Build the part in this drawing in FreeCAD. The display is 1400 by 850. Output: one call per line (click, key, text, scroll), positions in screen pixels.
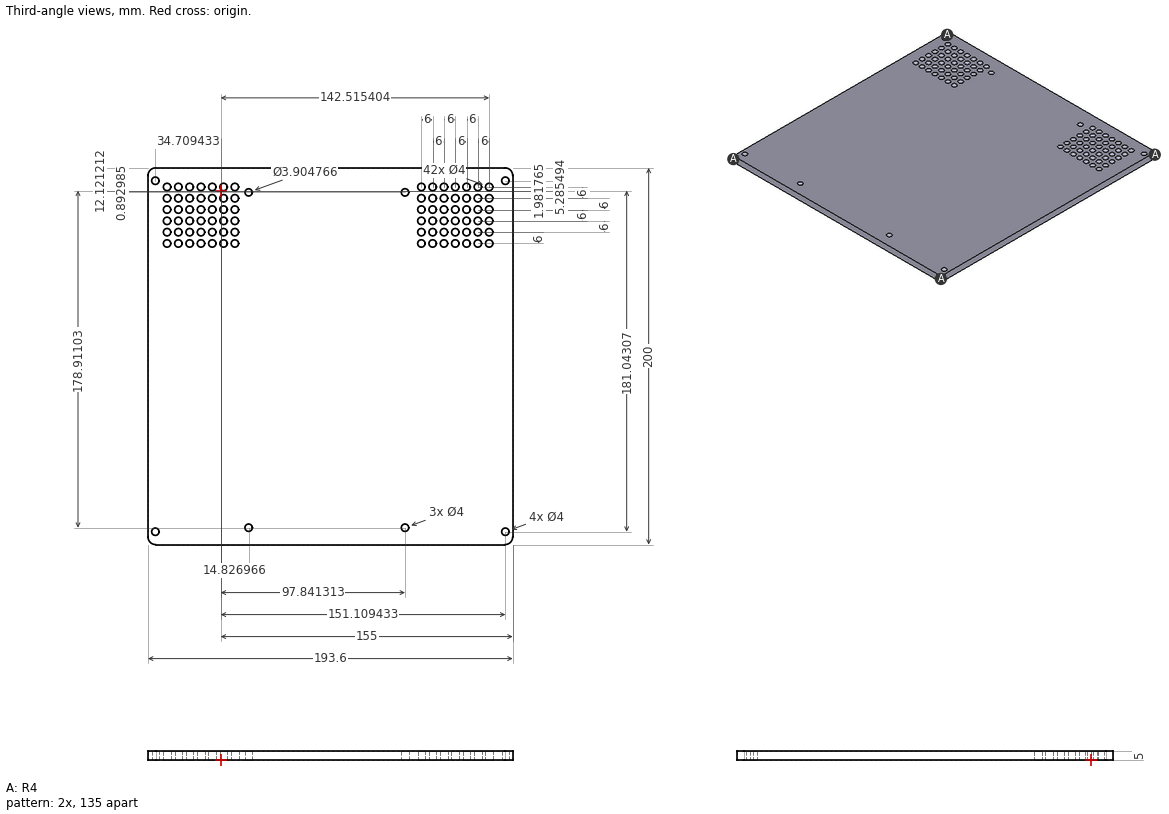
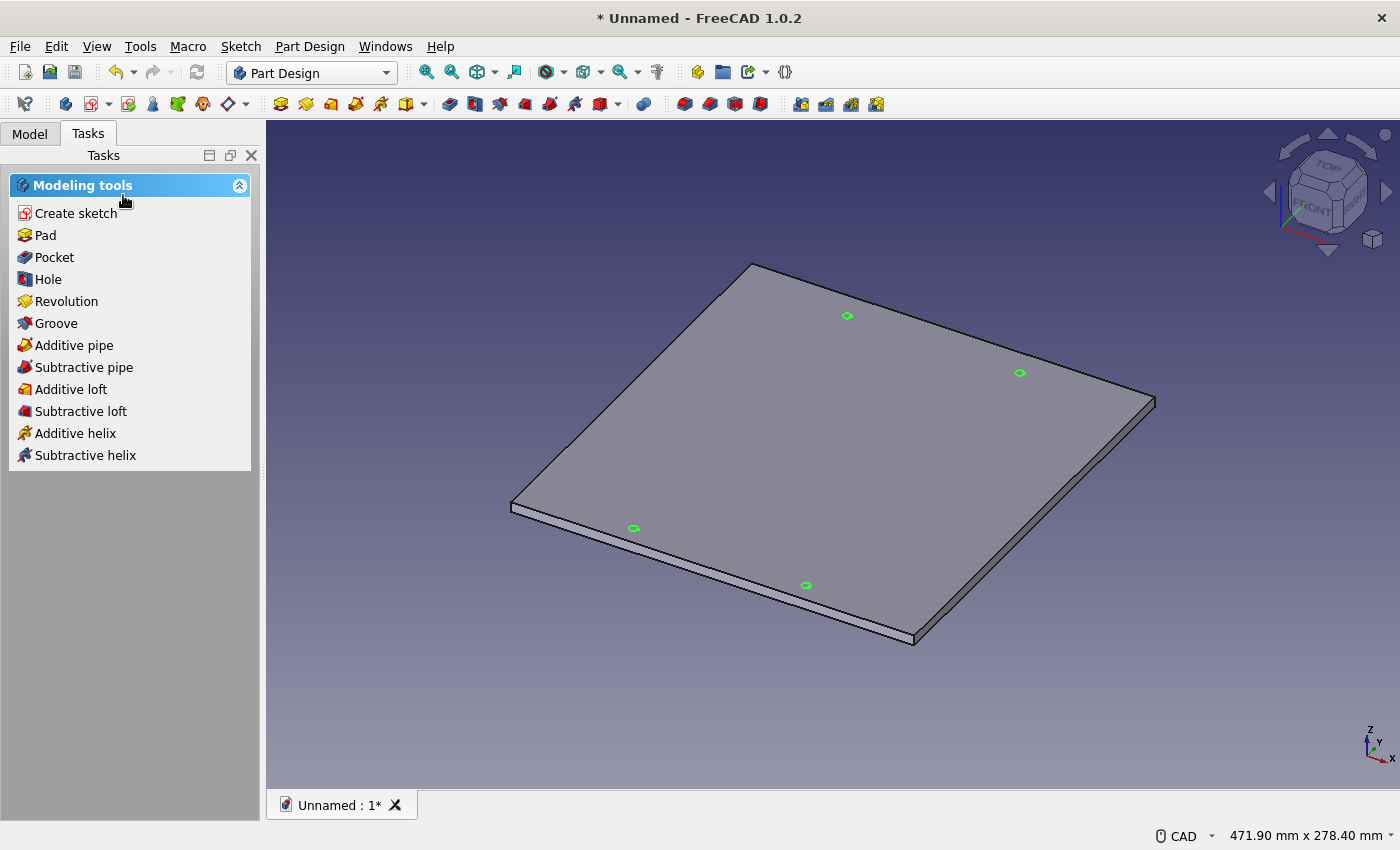
click(450, 104)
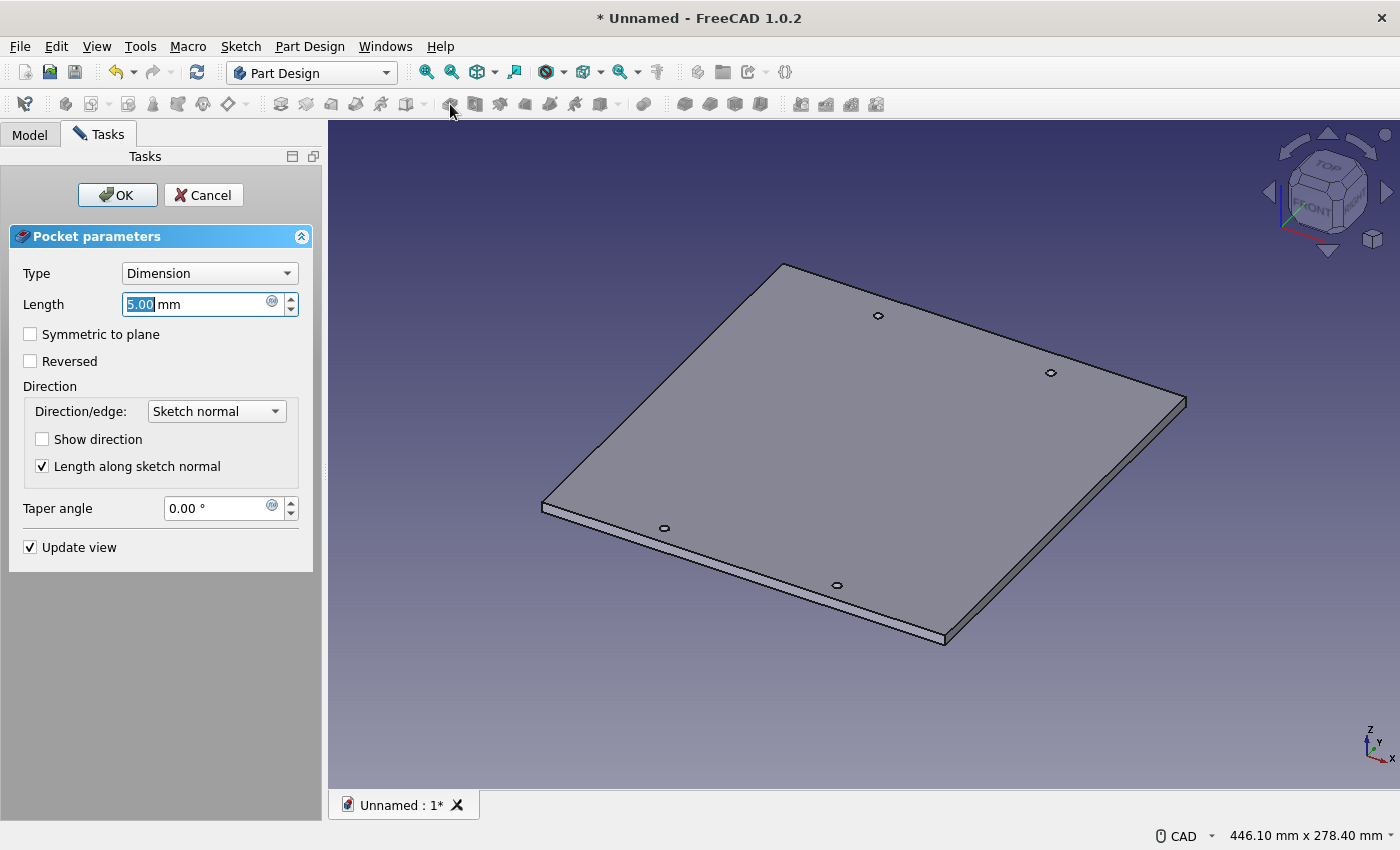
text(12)
key(Tab)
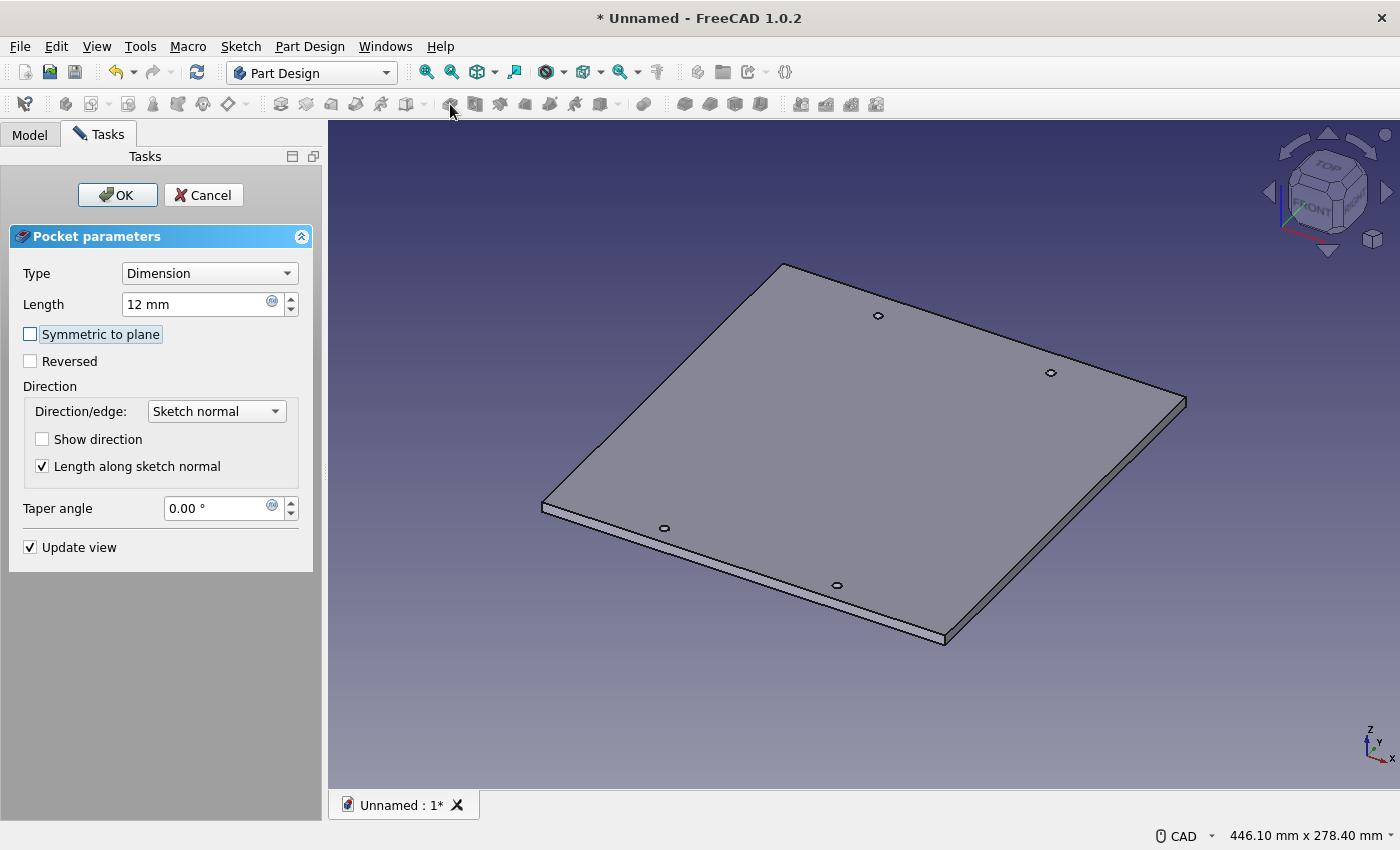
click(118, 195)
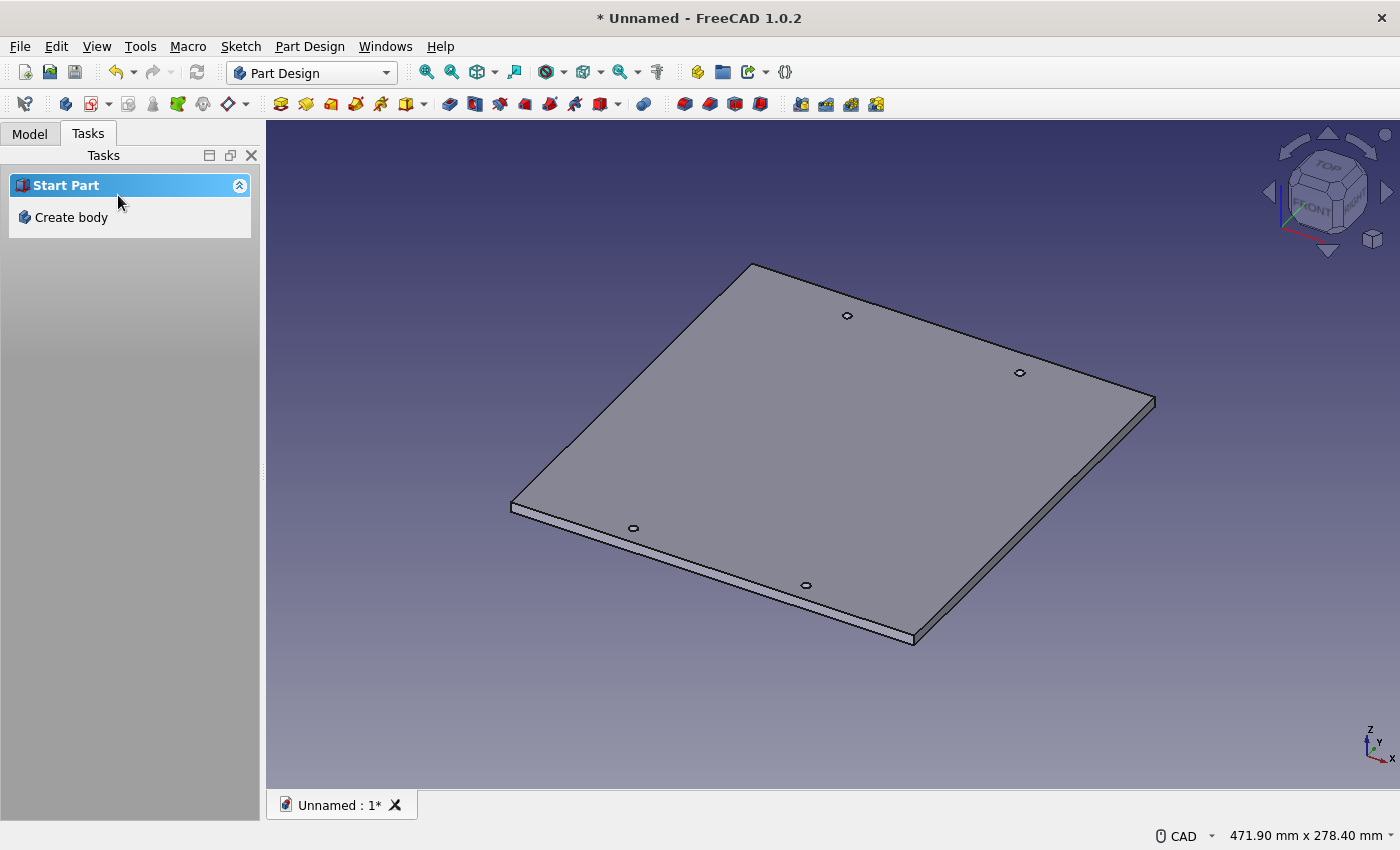
click(833, 449)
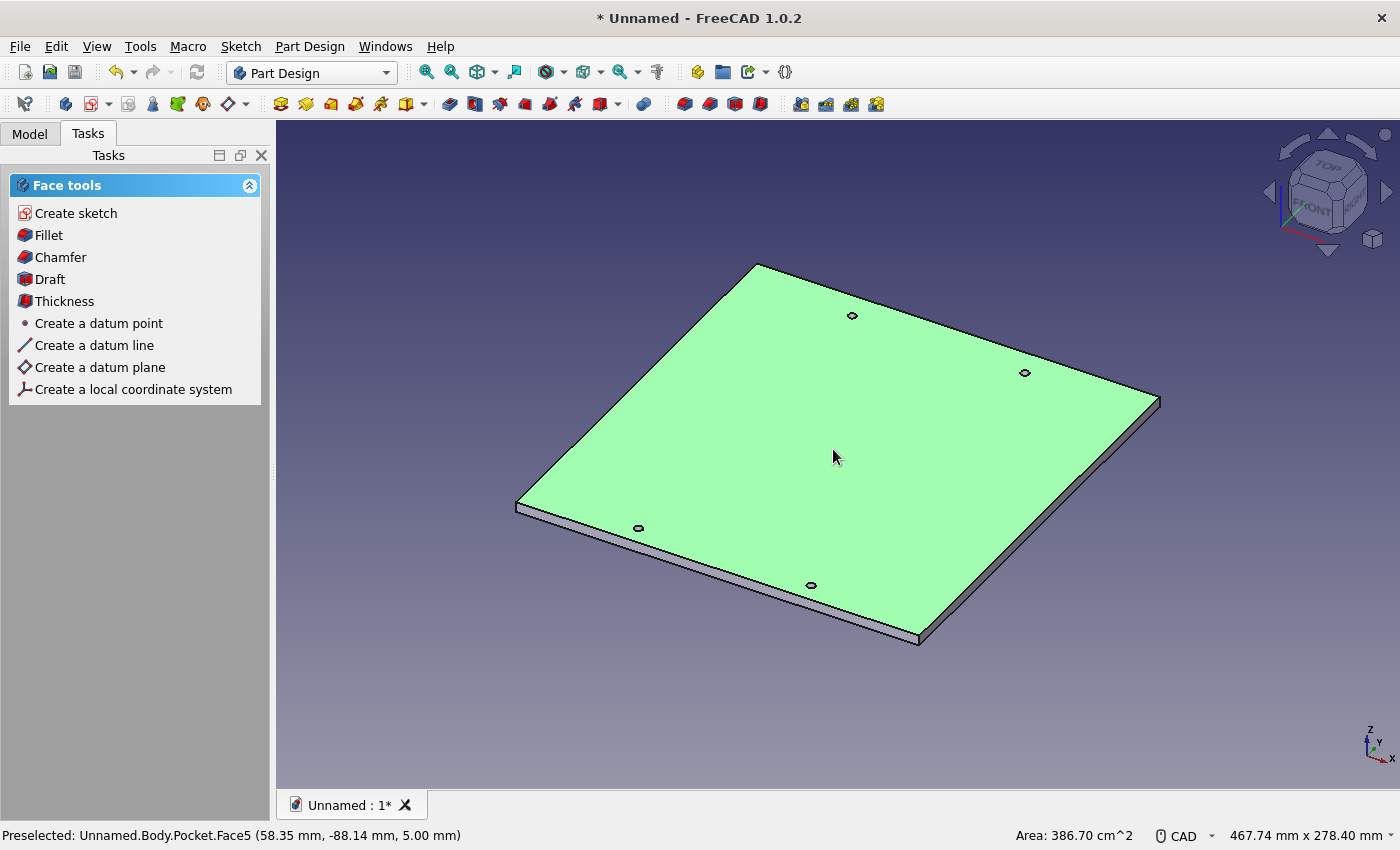
click(90, 104)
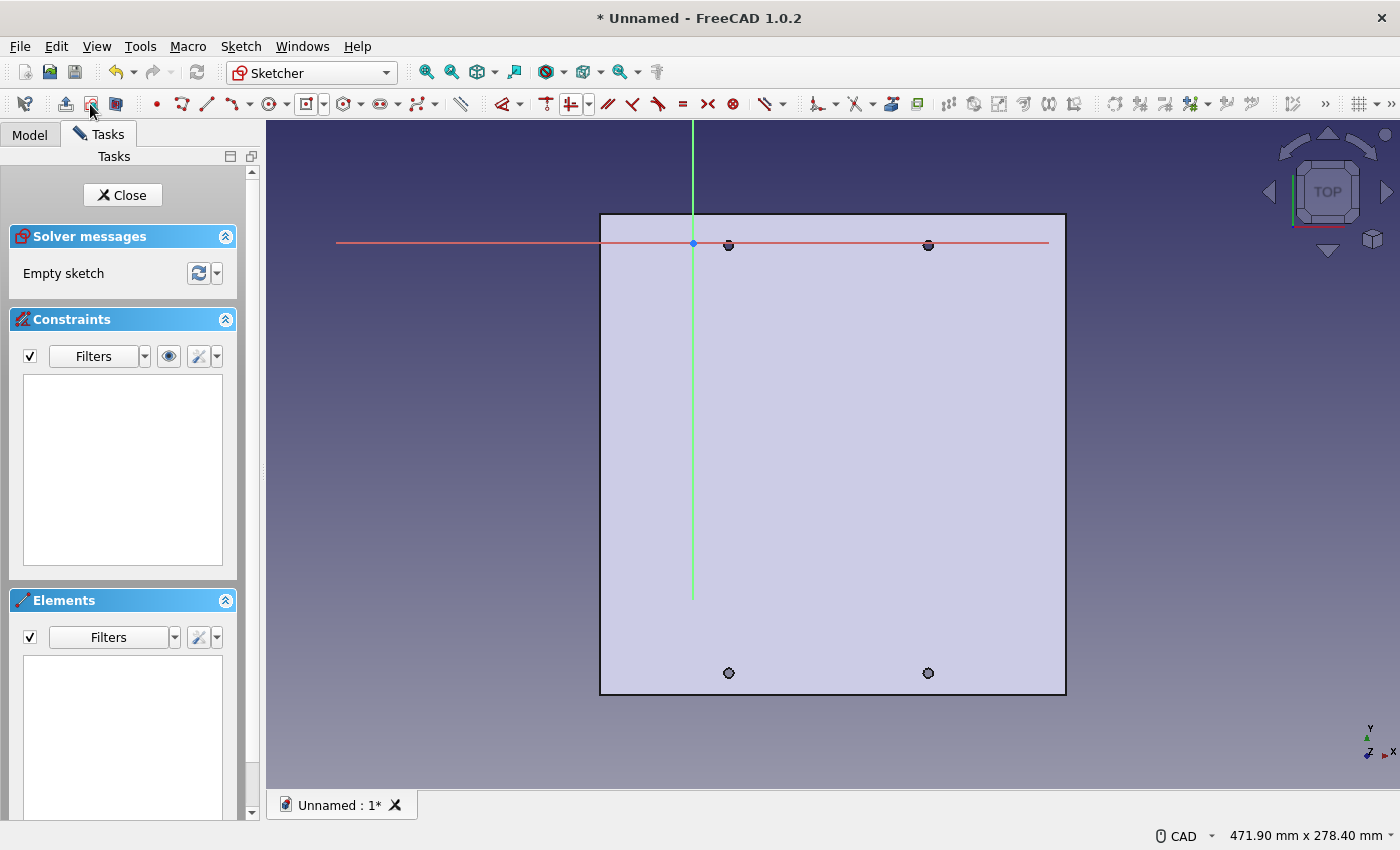
click(268, 104)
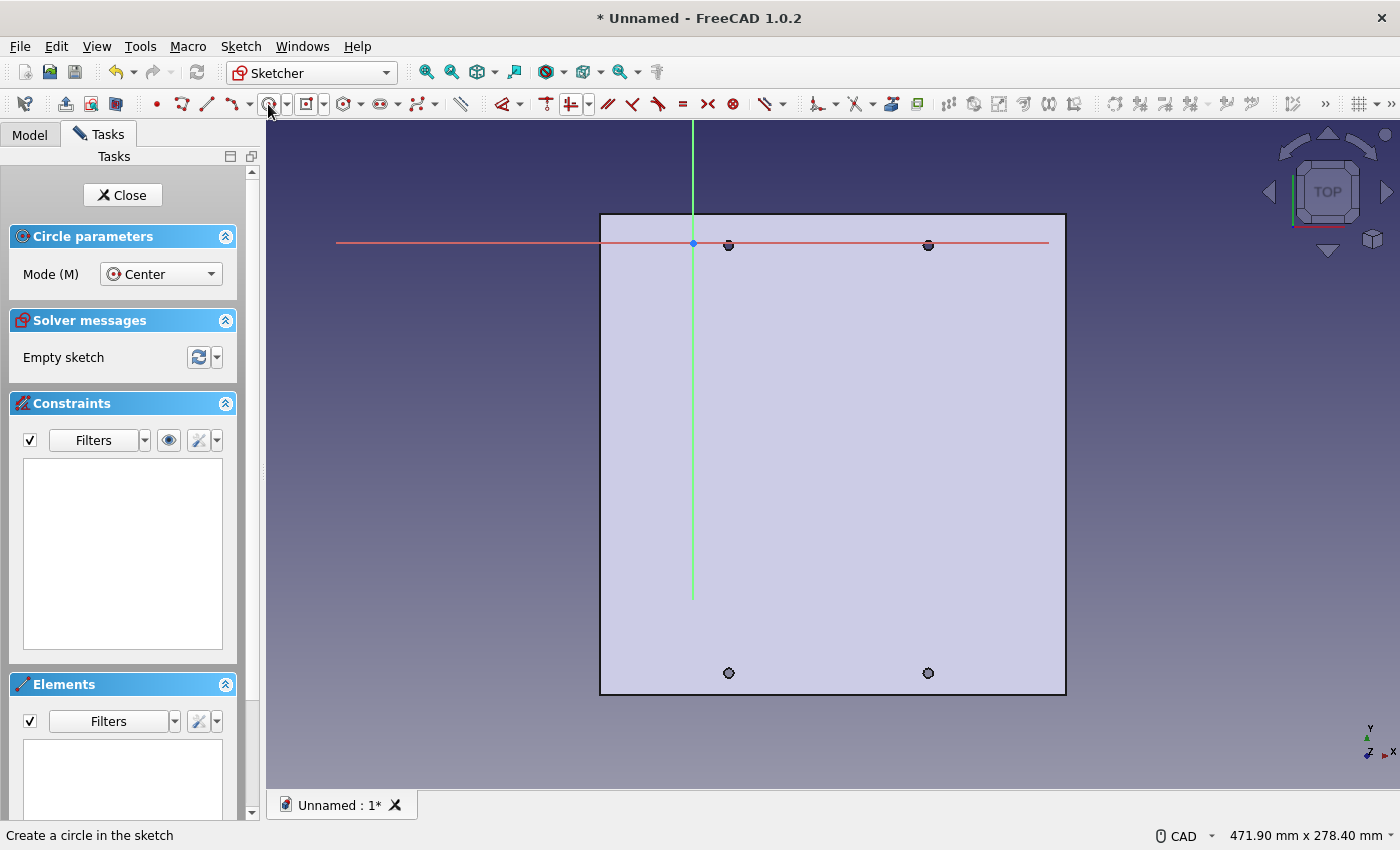
scroll(1056, 678, up, 8)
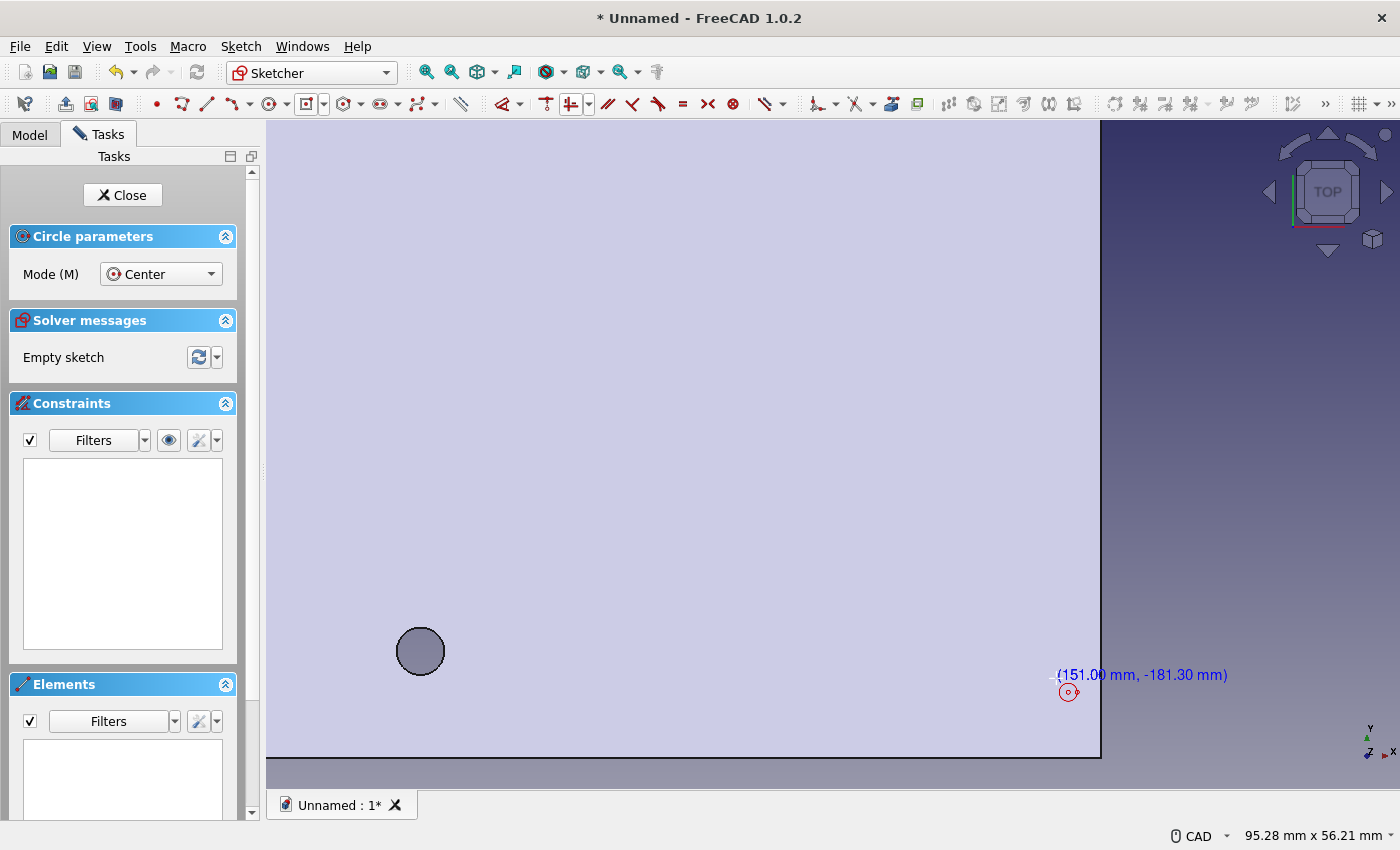
scroll(971, 679, down, 8)